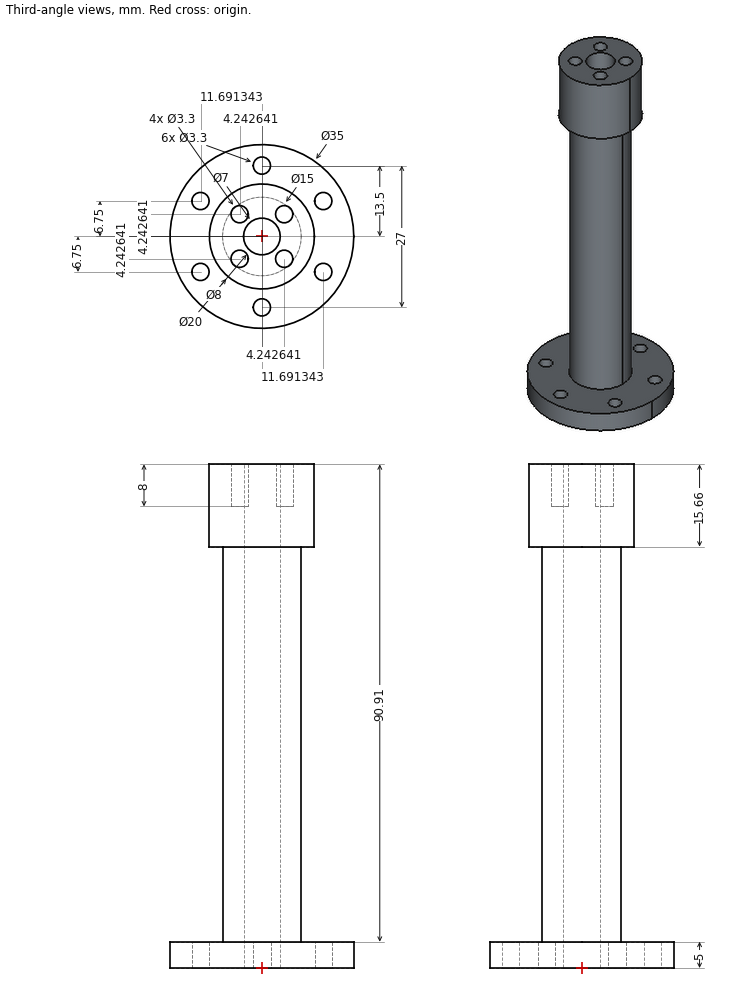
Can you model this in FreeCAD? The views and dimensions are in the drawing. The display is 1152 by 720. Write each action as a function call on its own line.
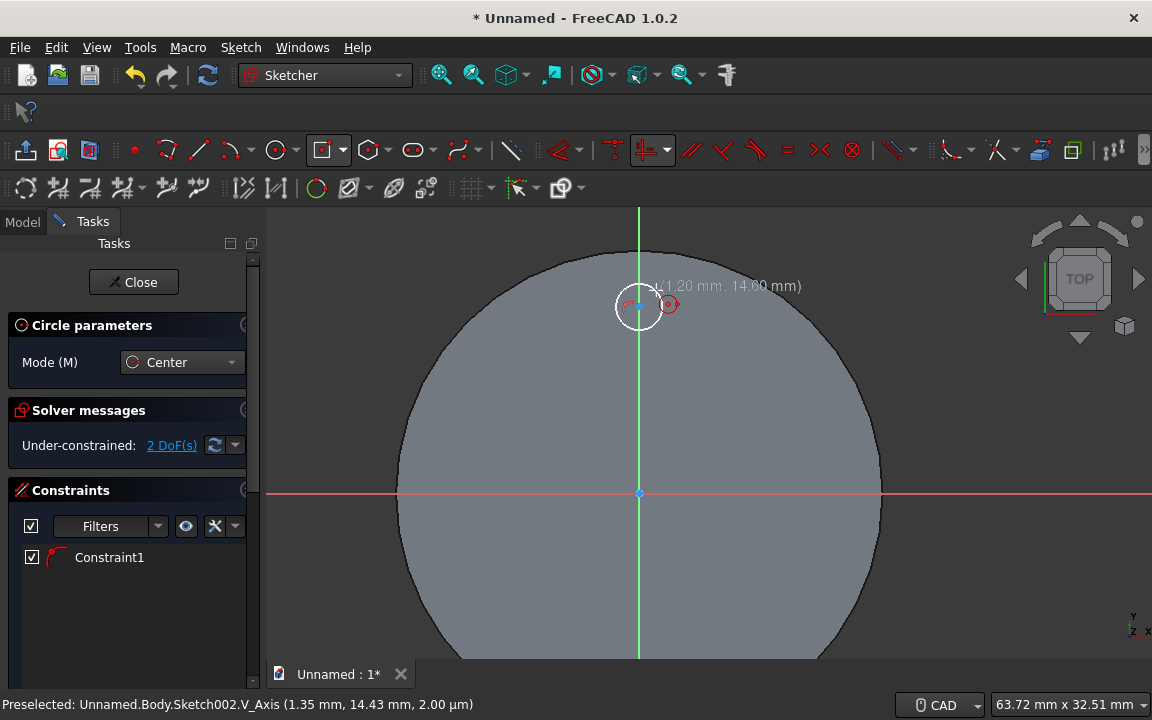
click(477, 400)
click(493, 384)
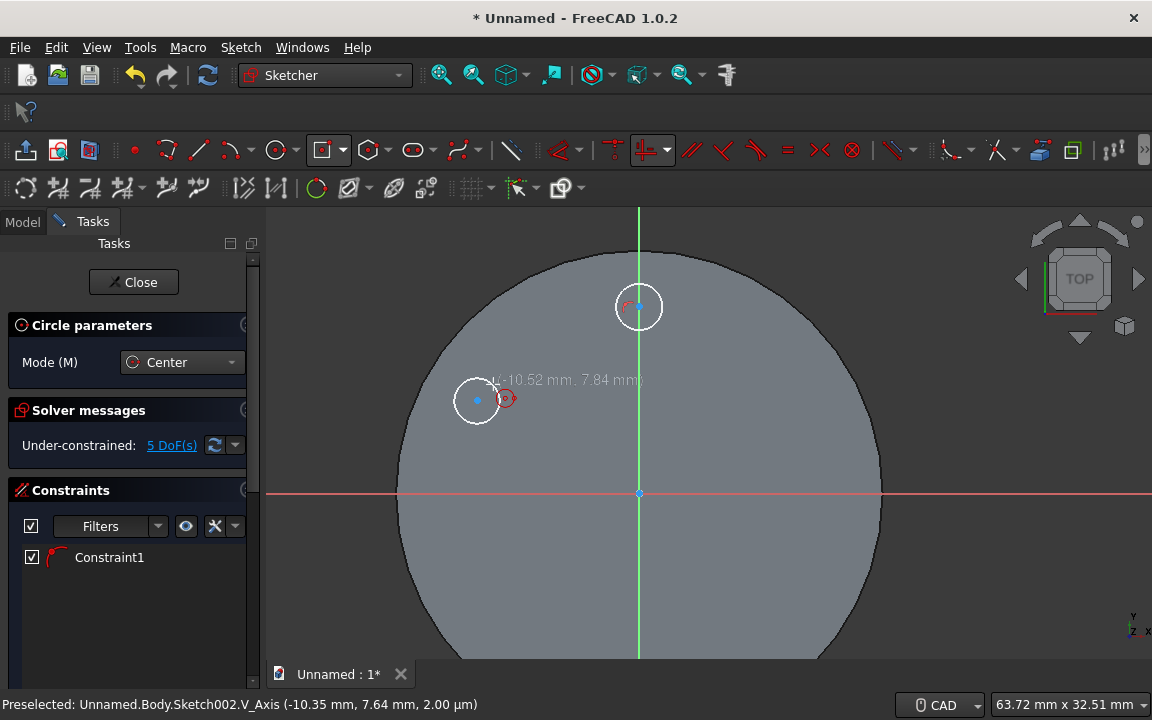
click(477, 588)
click(493, 572)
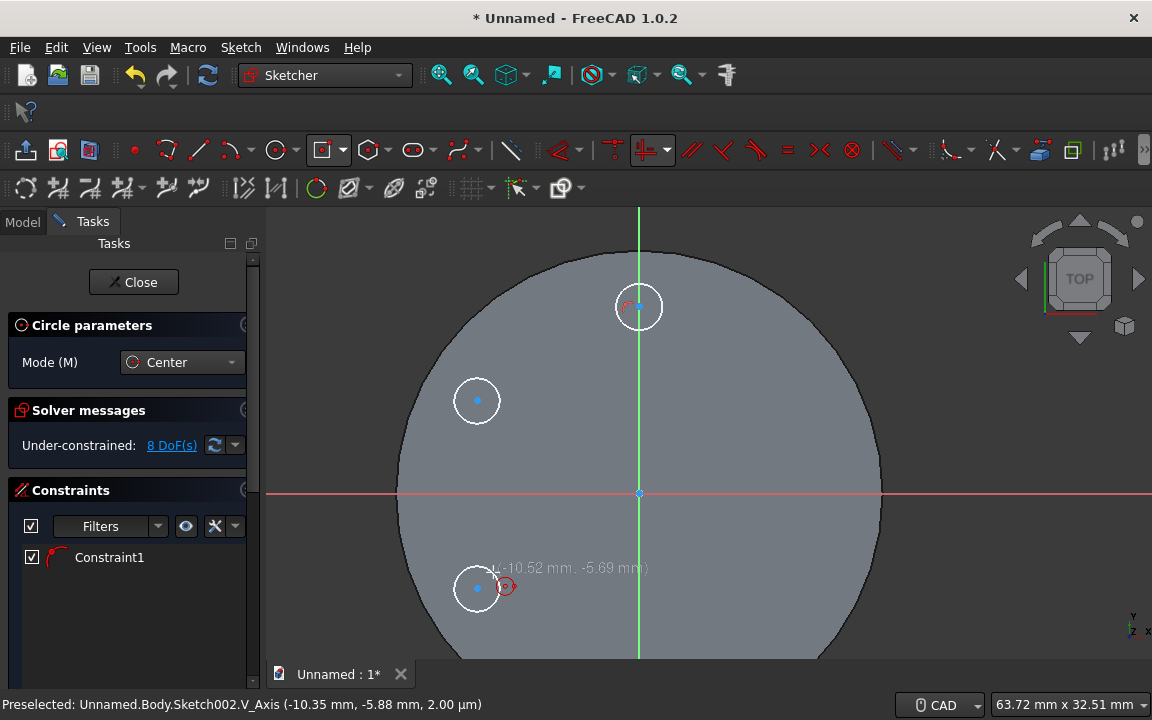
scroll(643, 309, down, 2)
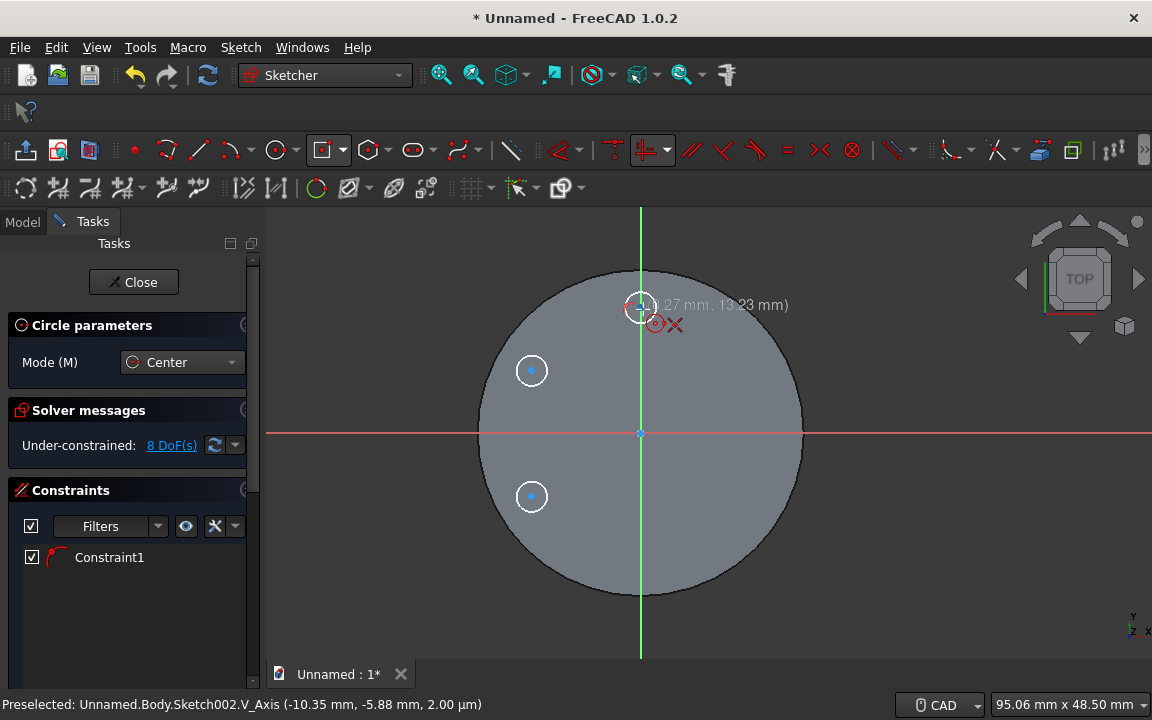
scroll(641, 559, up, 2)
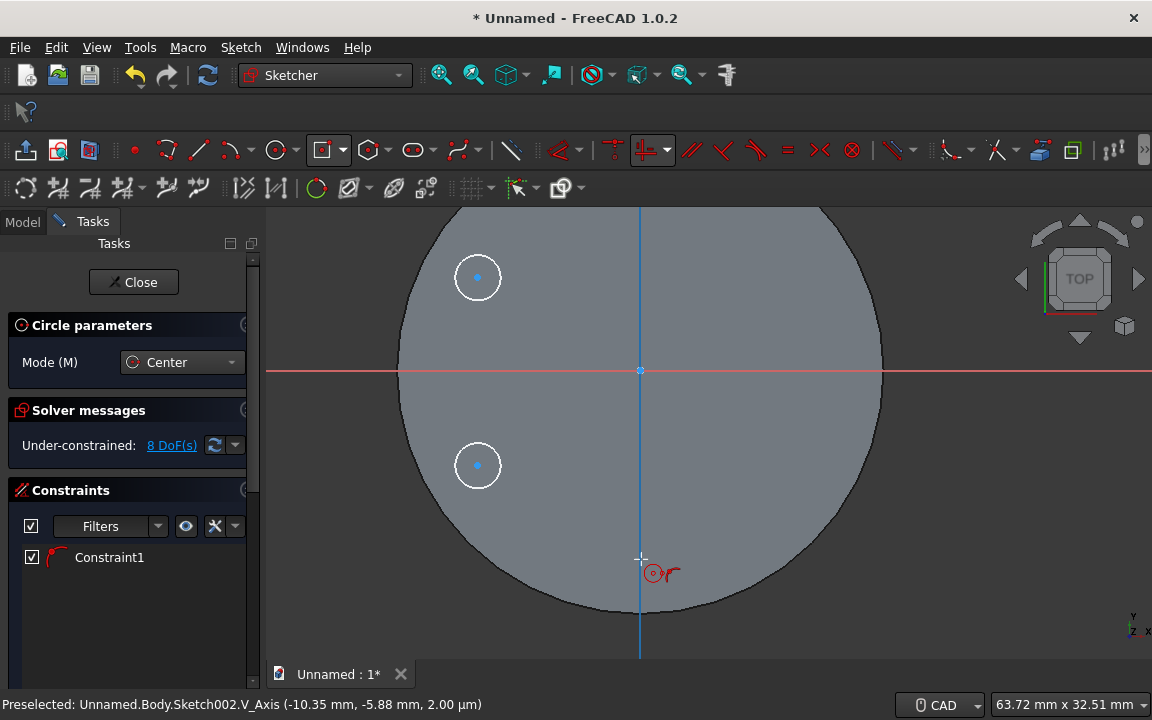
click(640, 558)
click(657, 542)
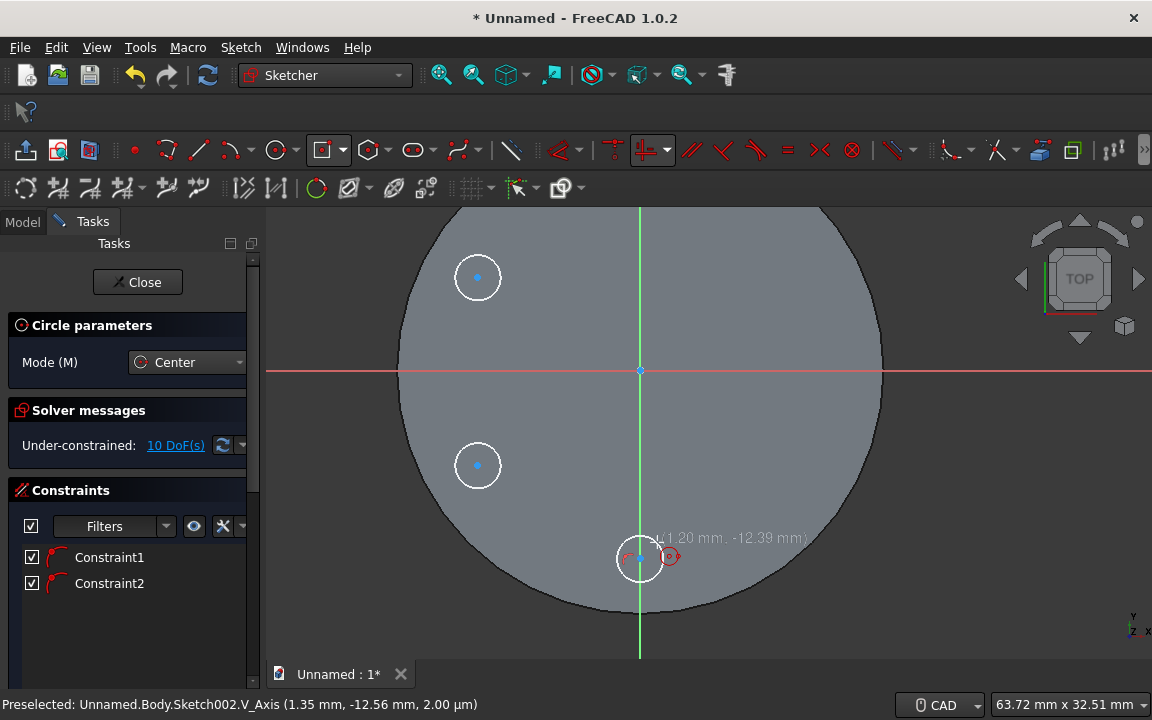
click(803, 465)
click(819, 448)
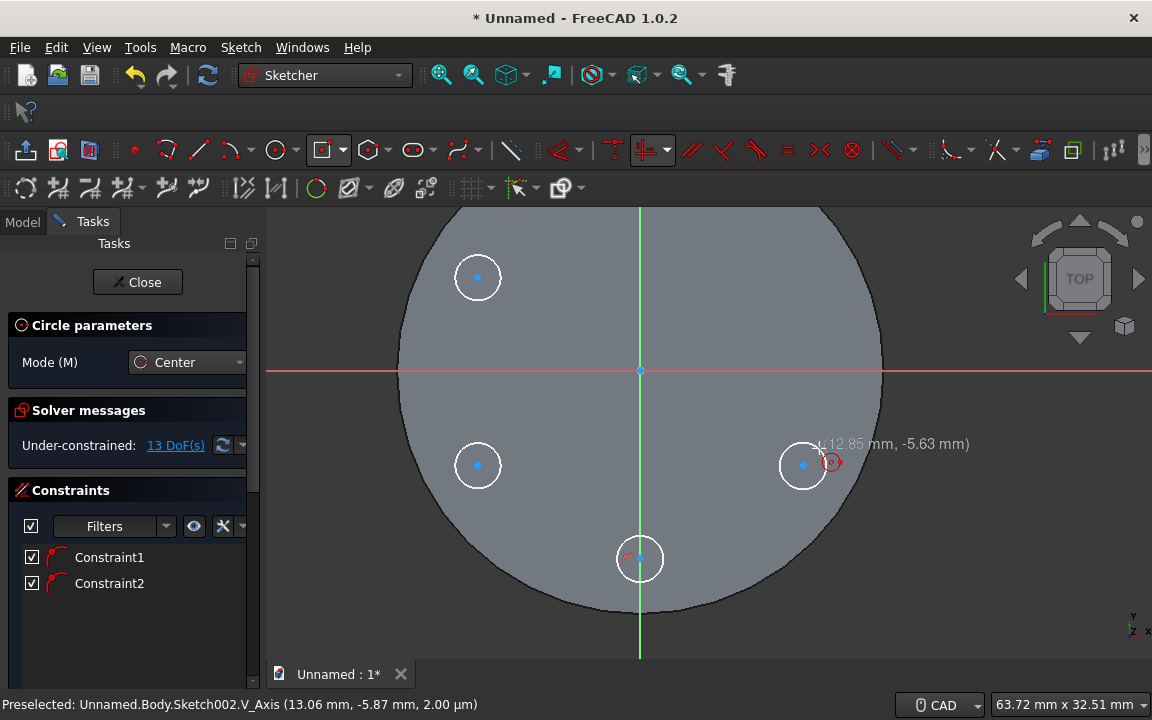
click(803, 277)
click(819, 261)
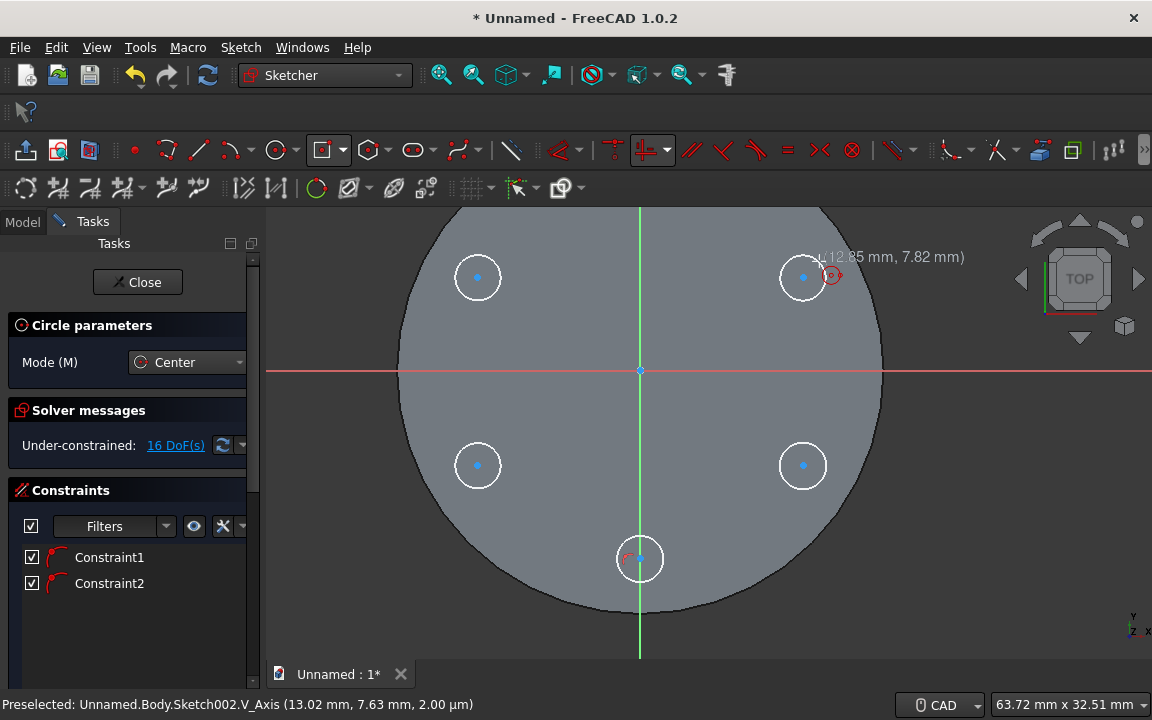
click(640, 371)
click(675, 336)
key(Escape)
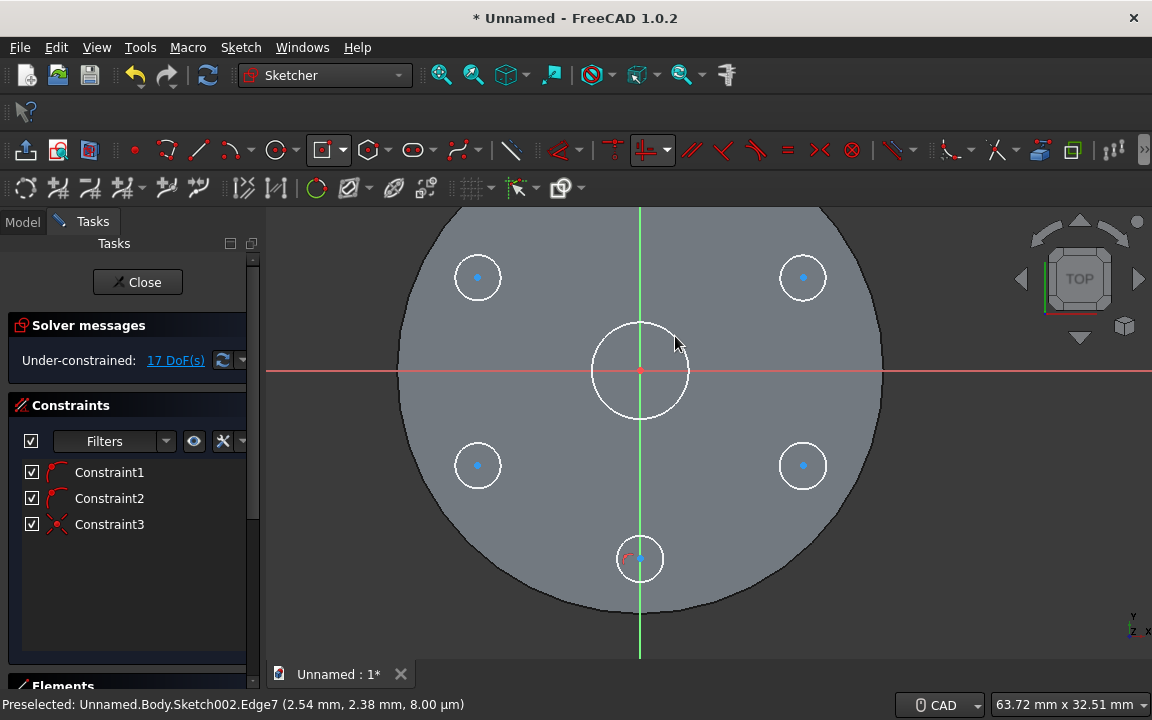
scroll(641, 560, down, 2)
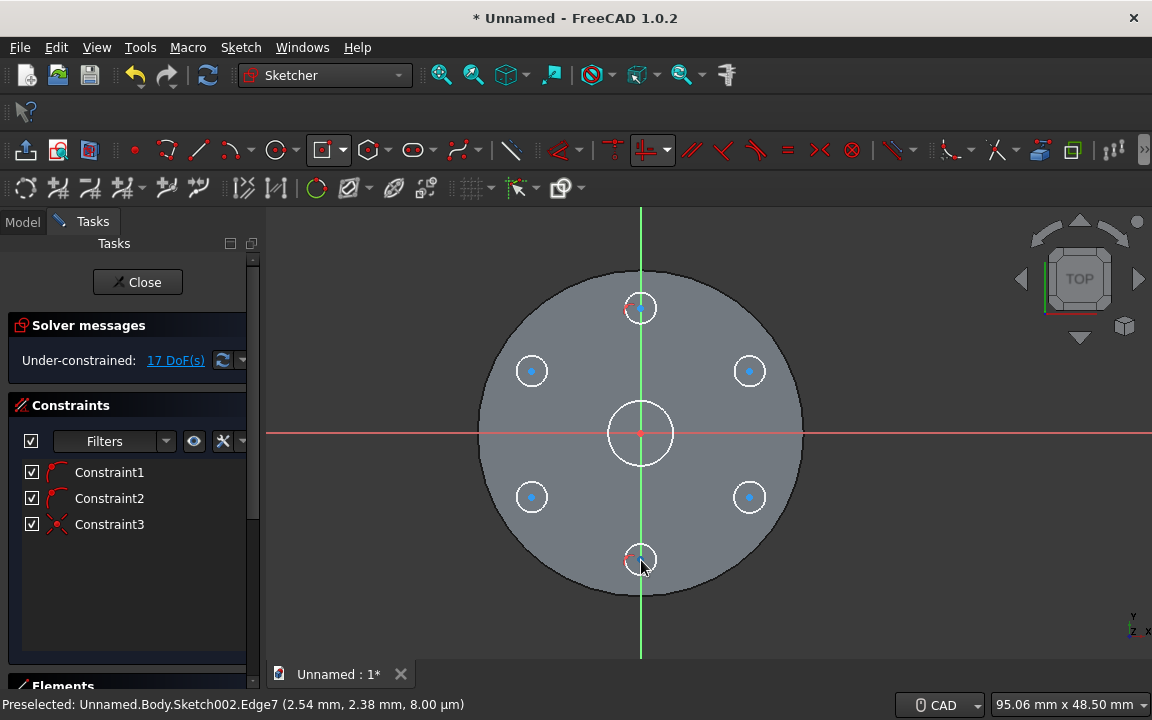
scroll(652, 297, up, 2)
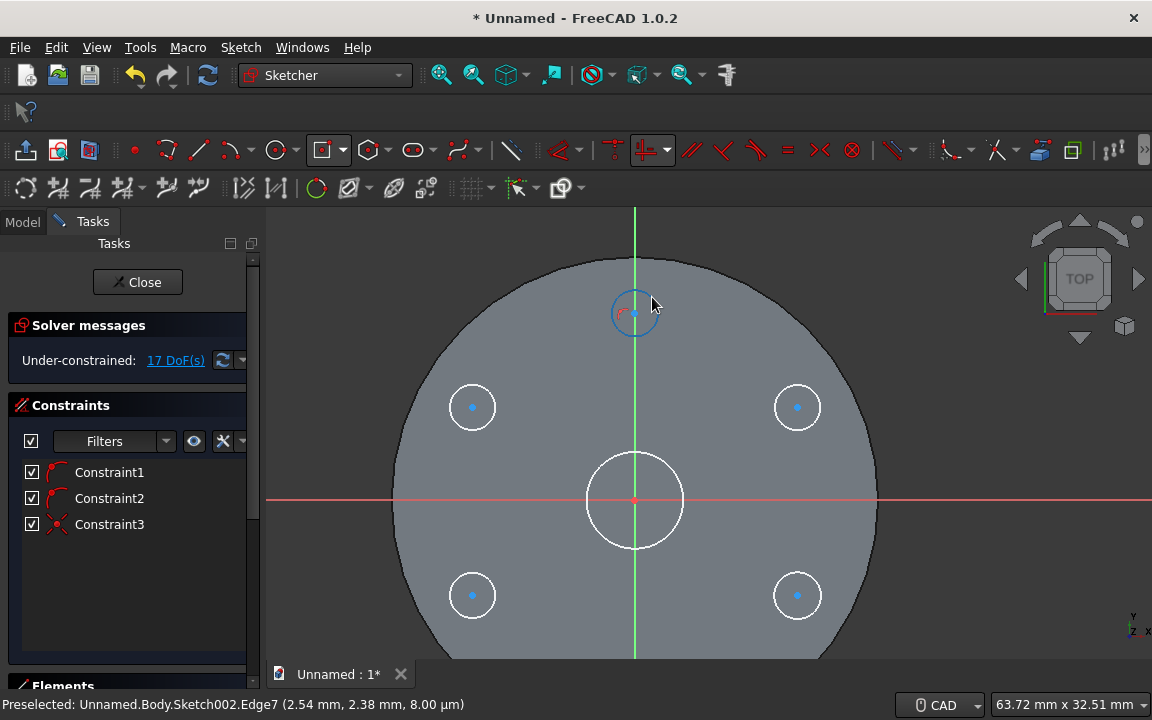
click(651, 297)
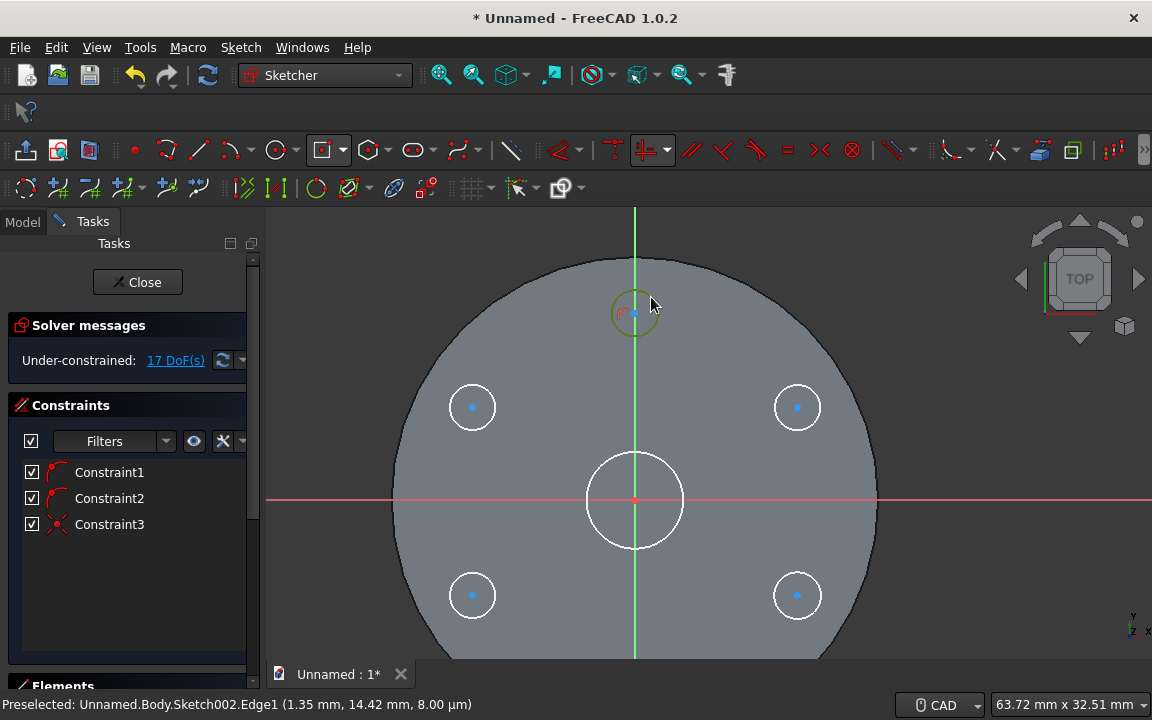
click(489, 391)